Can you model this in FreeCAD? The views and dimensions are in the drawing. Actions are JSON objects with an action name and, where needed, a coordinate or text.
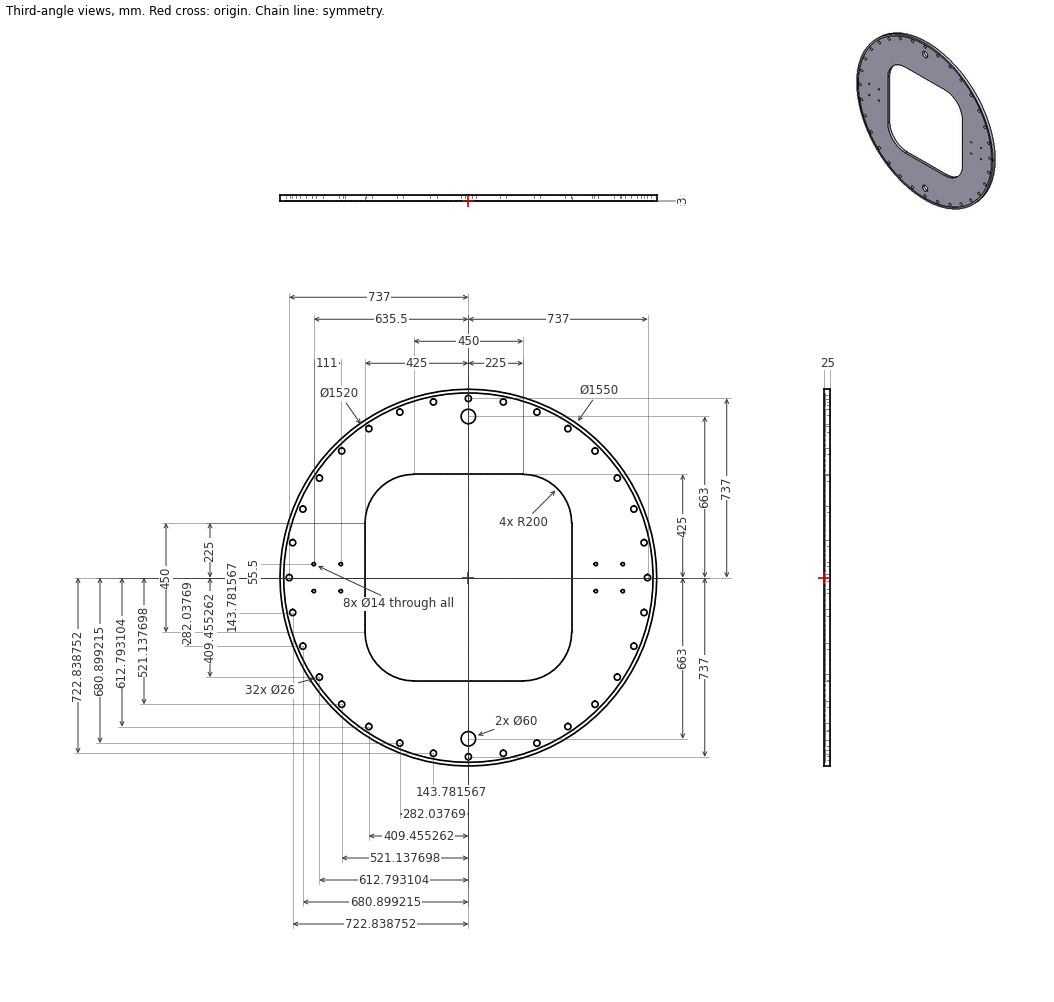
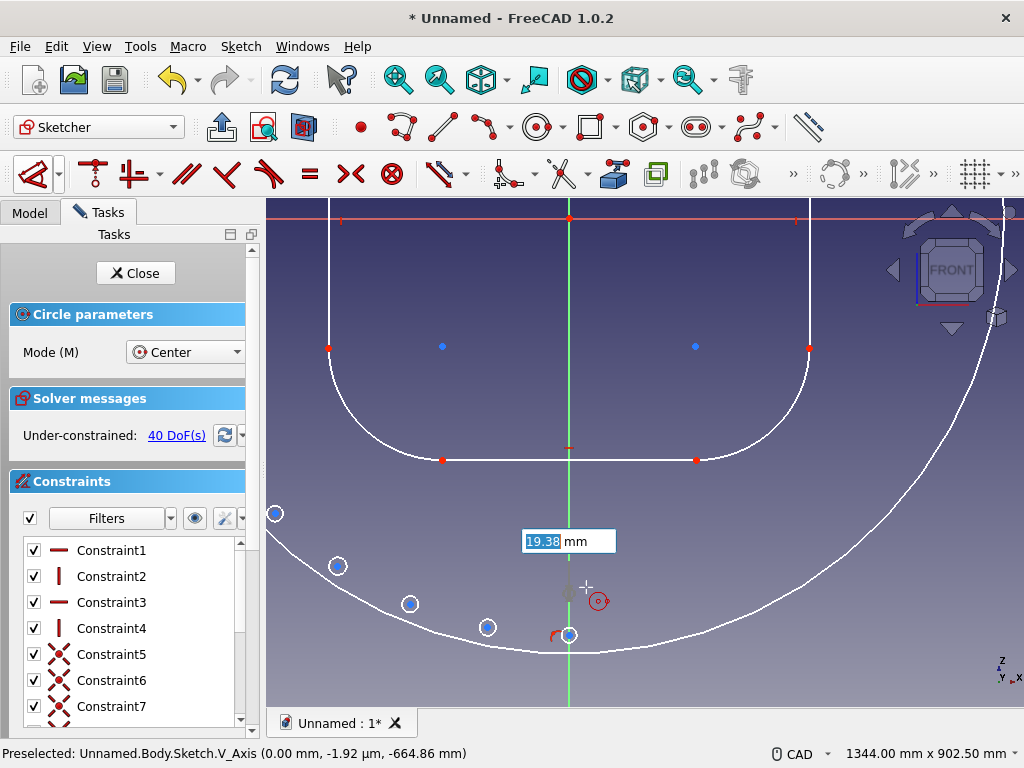
{"action": "left_click", "coordinate": [585, 587]}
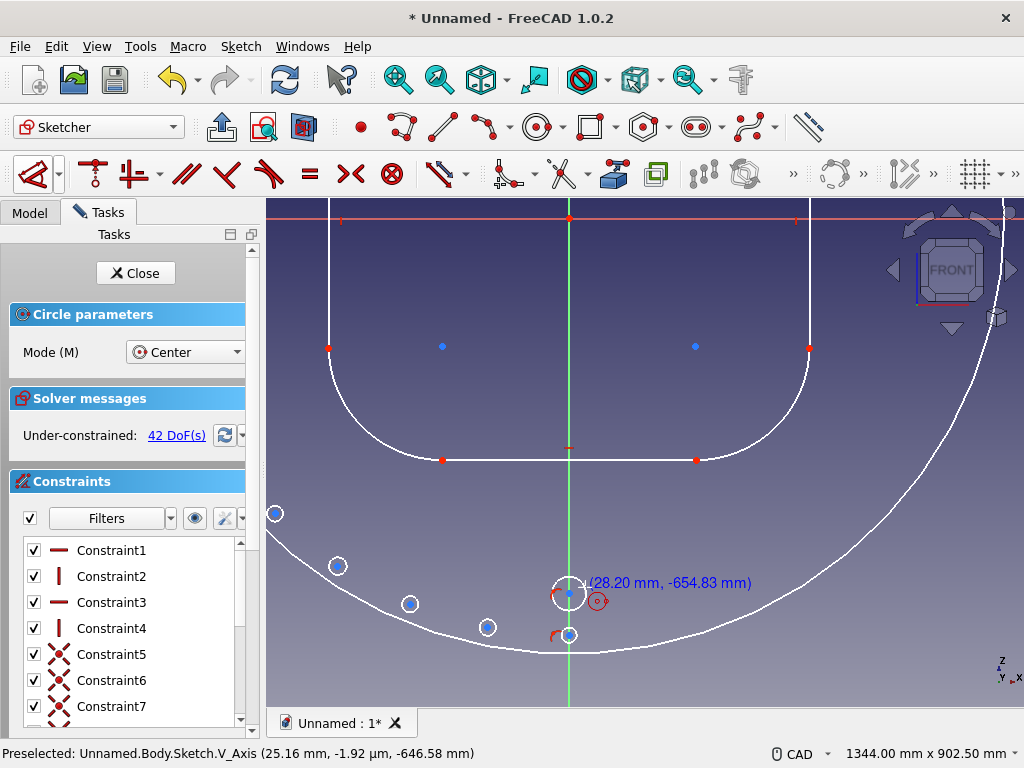
{"action": "scroll", "coordinate": [581, 589], "scroll_direction": "down", "scroll_amount": 5}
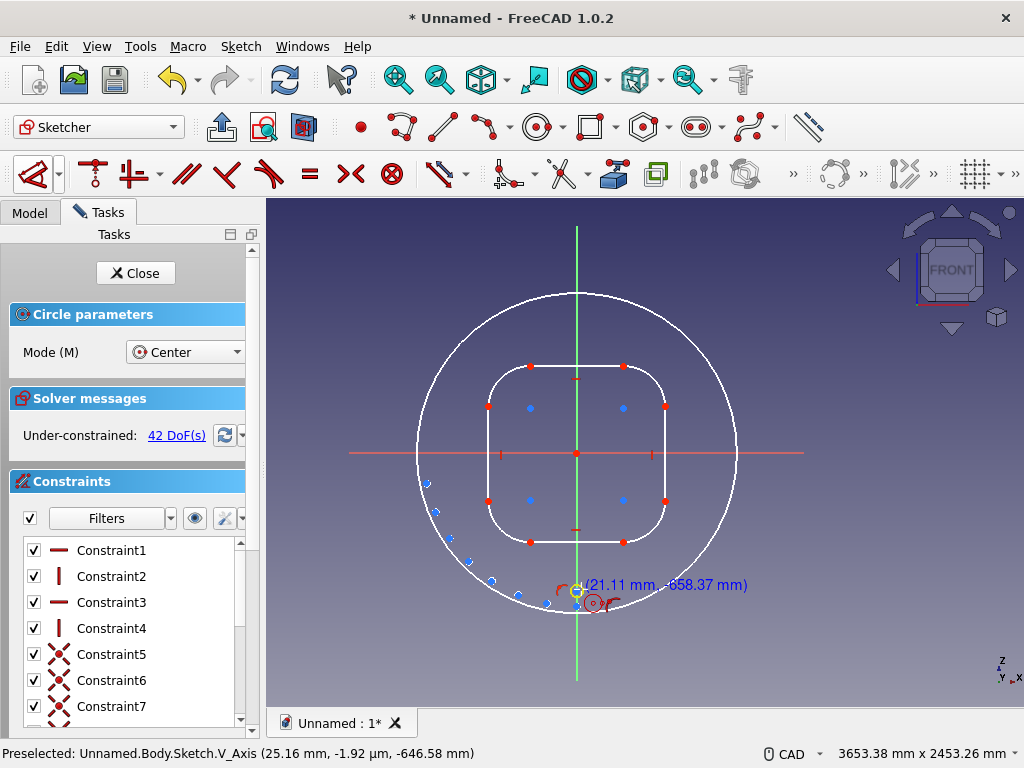
{"action": "scroll", "coordinate": [424, 453], "scroll_direction": "up", "scroll_amount": 11}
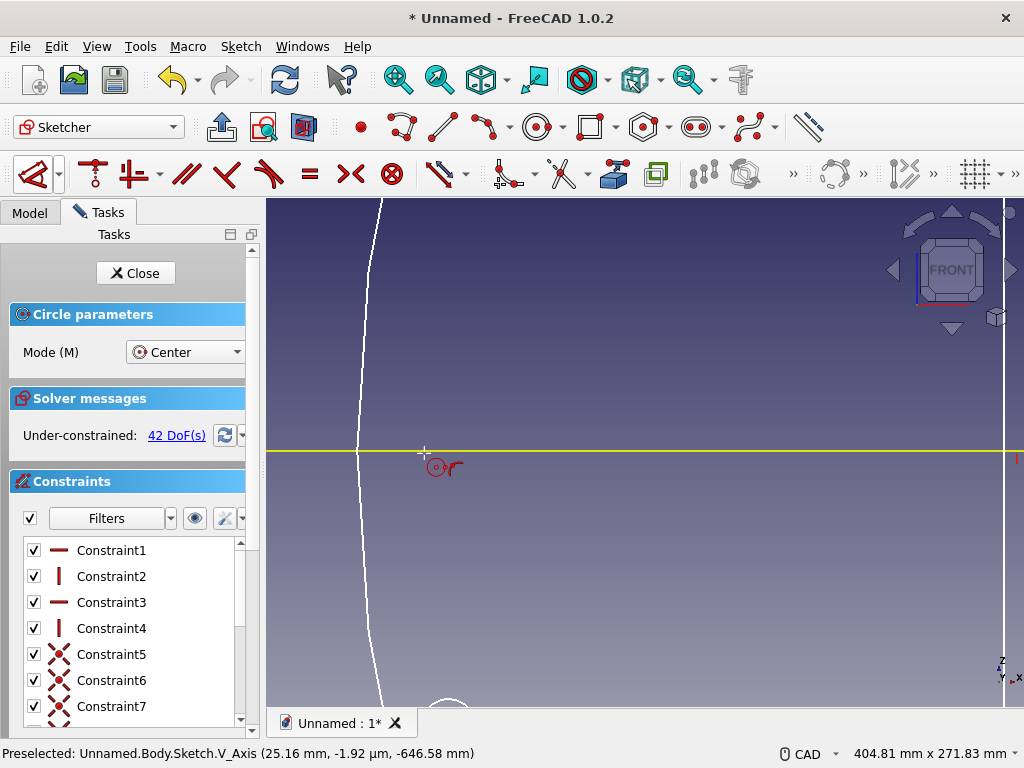
{"action": "scroll", "coordinate": [424, 453], "scroll_direction": "down", "scroll_amount": 11}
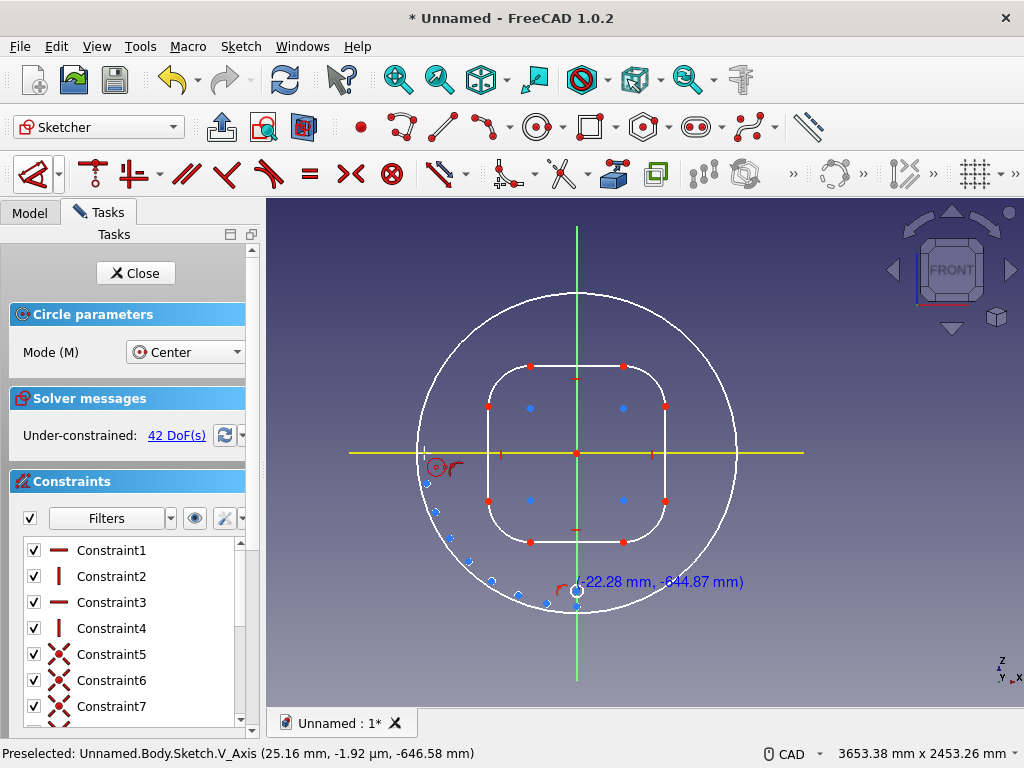
{"action": "scroll", "coordinate": [424, 453], "scroll_direction": "up", "scroll_amount": 4}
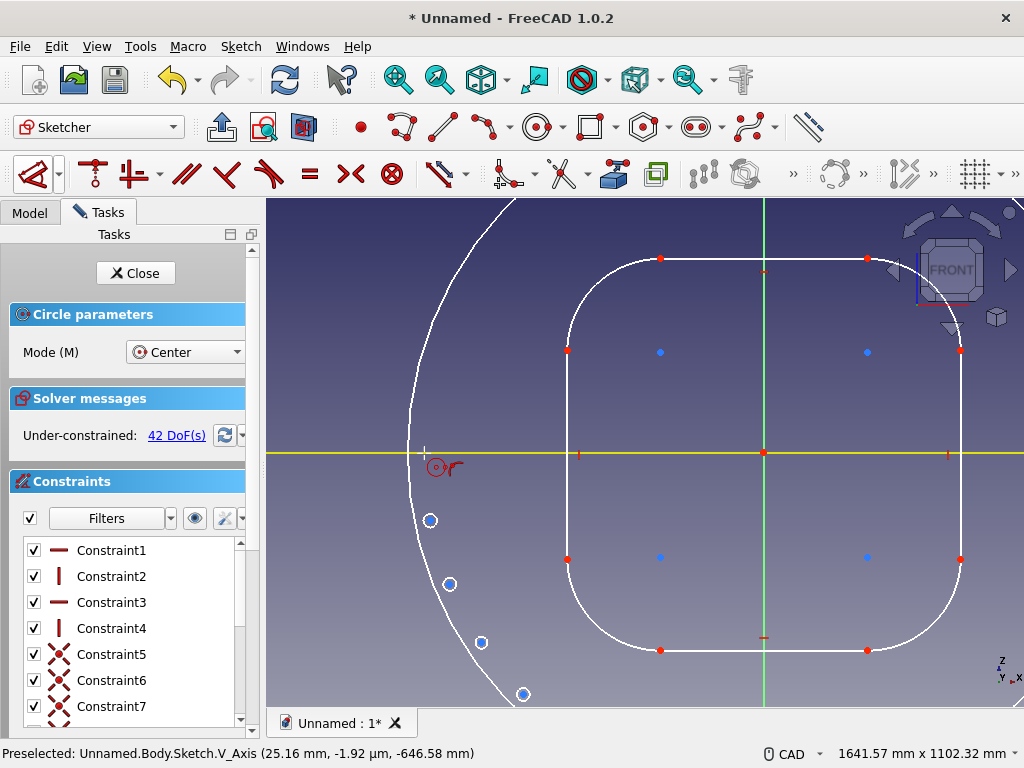
{"action": "left_click", "coordinate": [424, 453]}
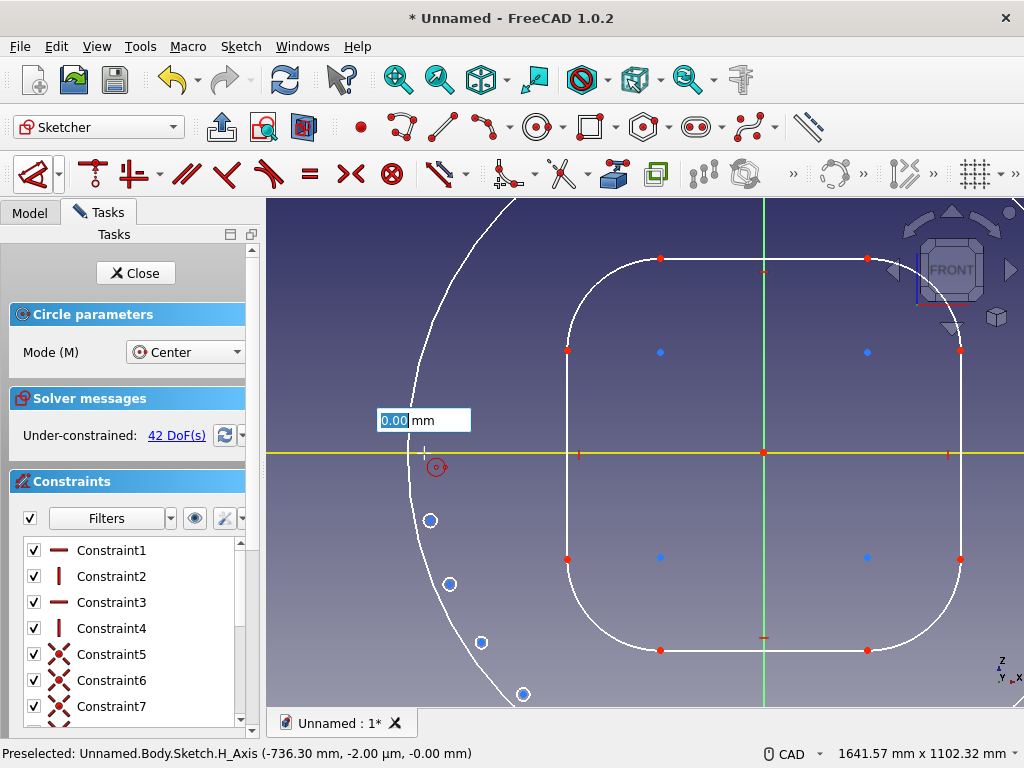
{"action": "scroll", "coordinate": [422, 459], "scroll_direction": "up", "scroll_amount": 6}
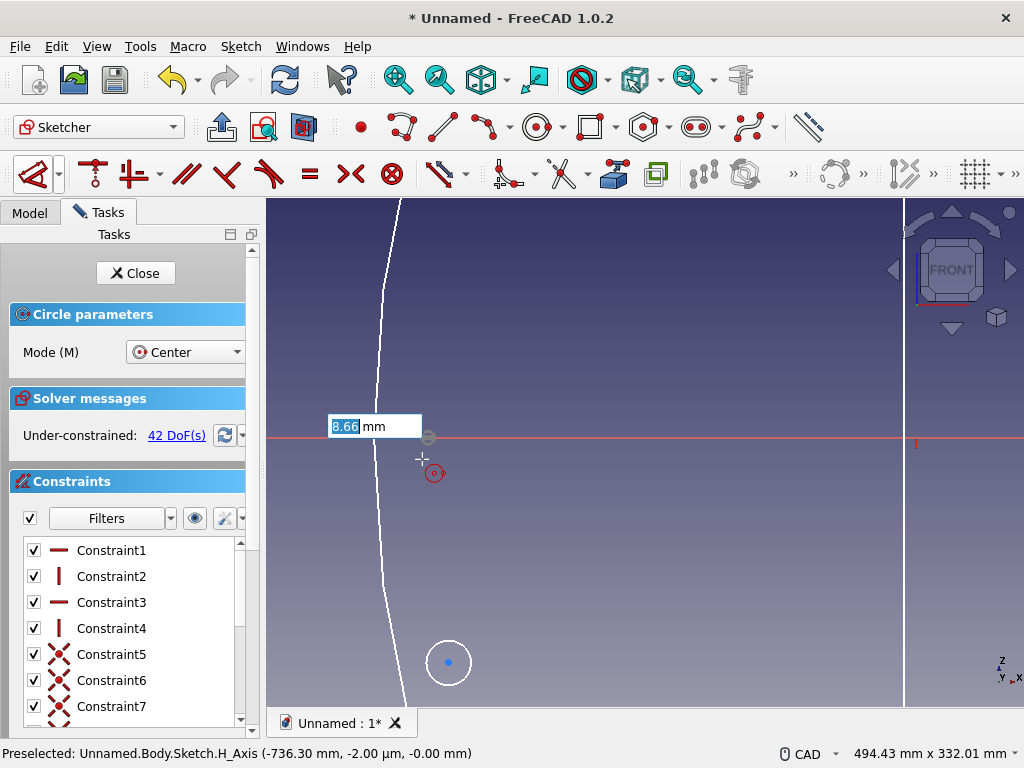
{"action": "left_click", "coordinate": [420, 456]}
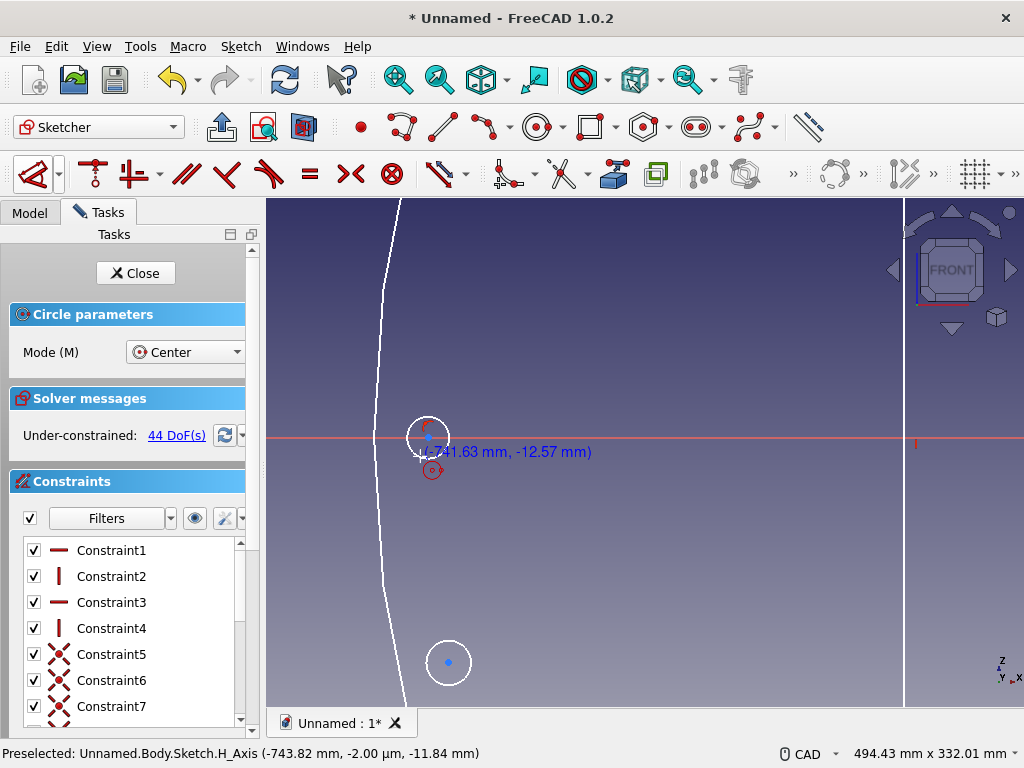
{"action": "scroll", "coordinate": [423, 455], "scroll_direction": "down", "scroll_amount": 10}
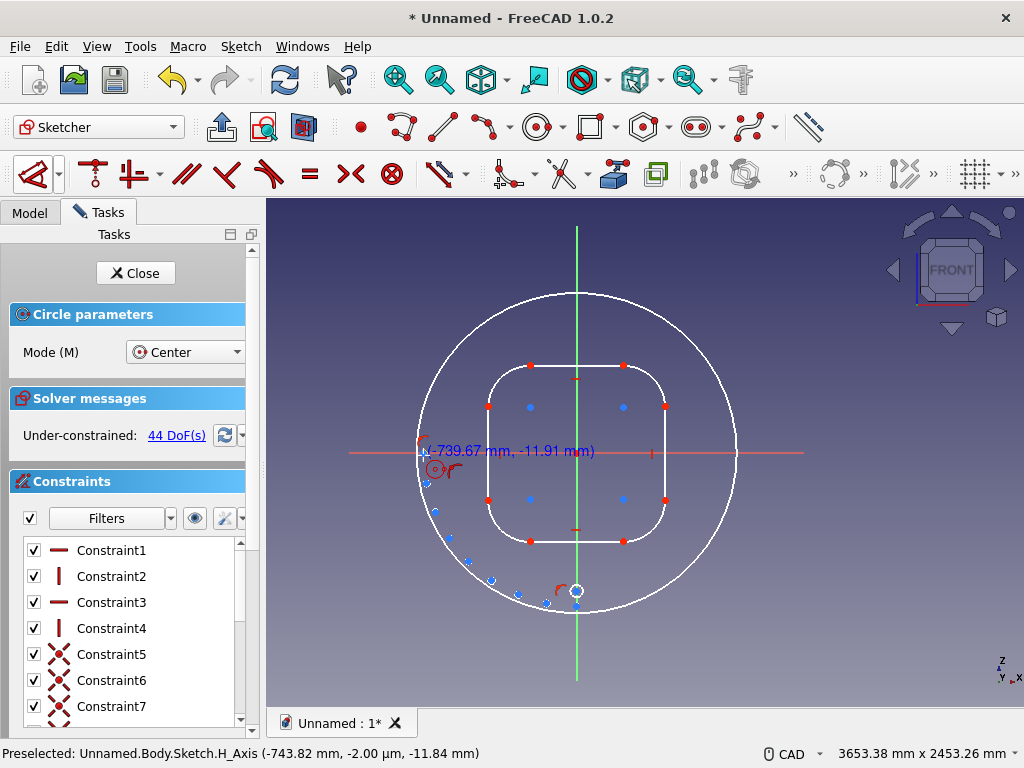
{"action": "scroll", "coordinate": [427, 423], "scroll_direction": "up", "scroll_amount": 11}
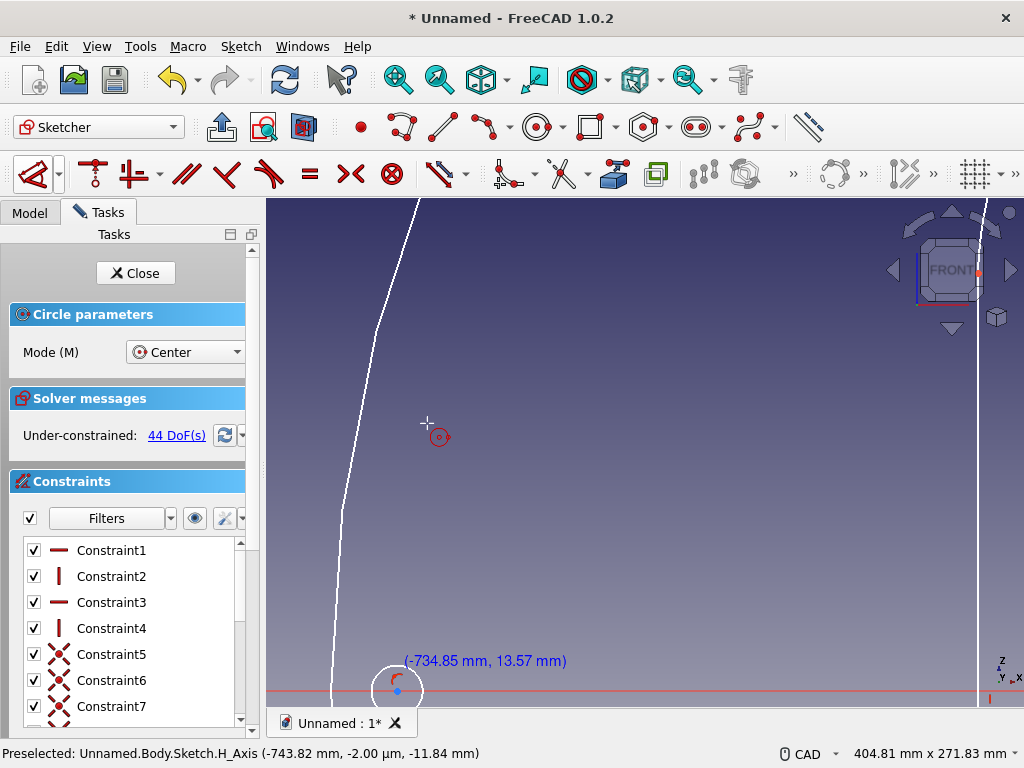
{"action": "scroll", "coordinate": [427, 423], "scroll_direction": "down", "scroll_amount": 11}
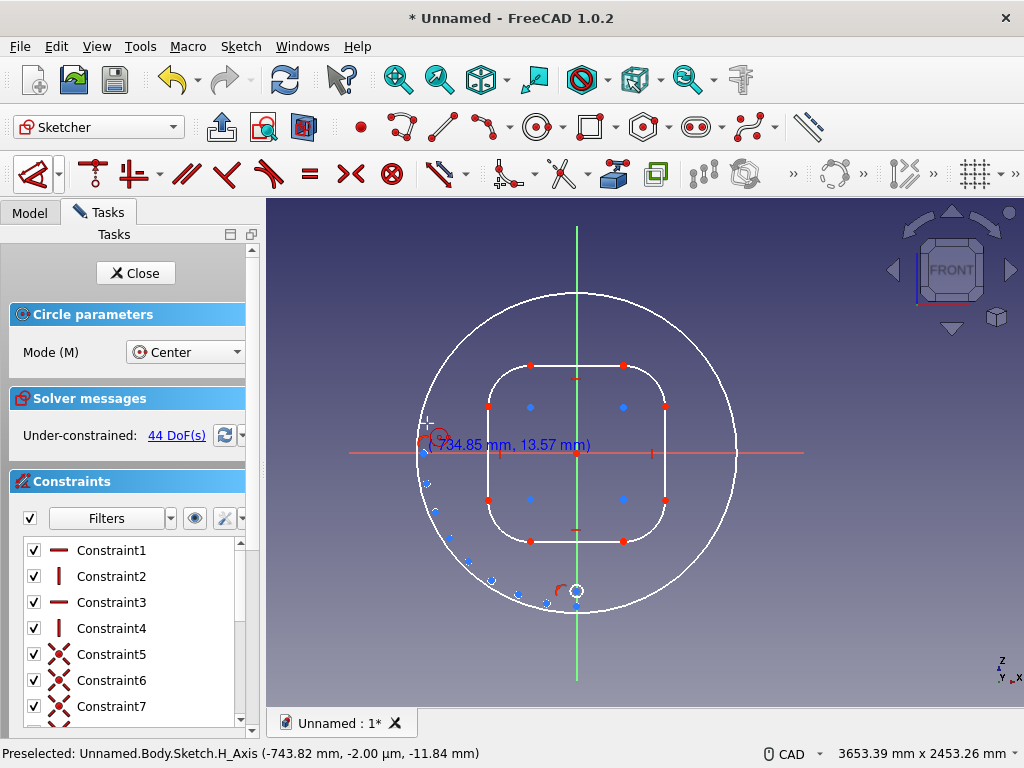
{"action": "scroll", "coordinate": [427, 423], "scroll_direction": "up", "scroll_amount": 4}